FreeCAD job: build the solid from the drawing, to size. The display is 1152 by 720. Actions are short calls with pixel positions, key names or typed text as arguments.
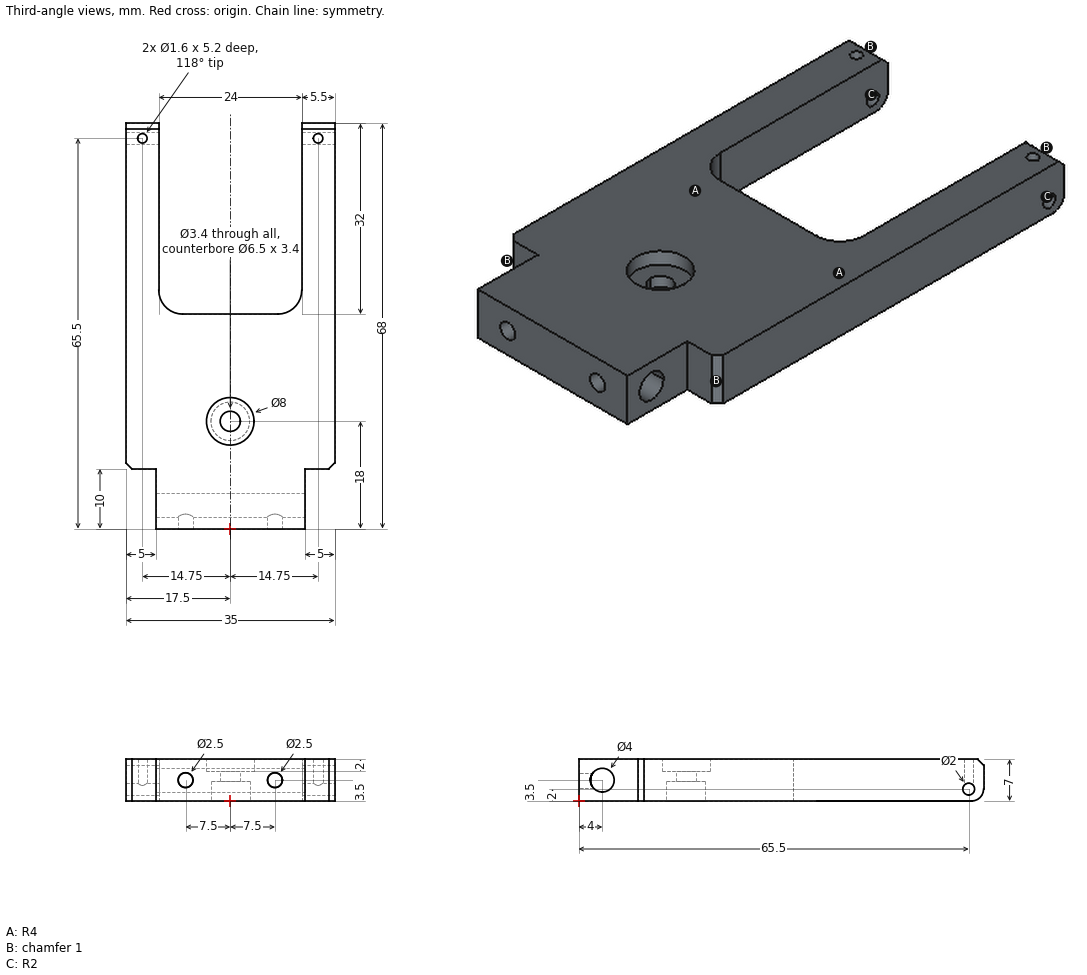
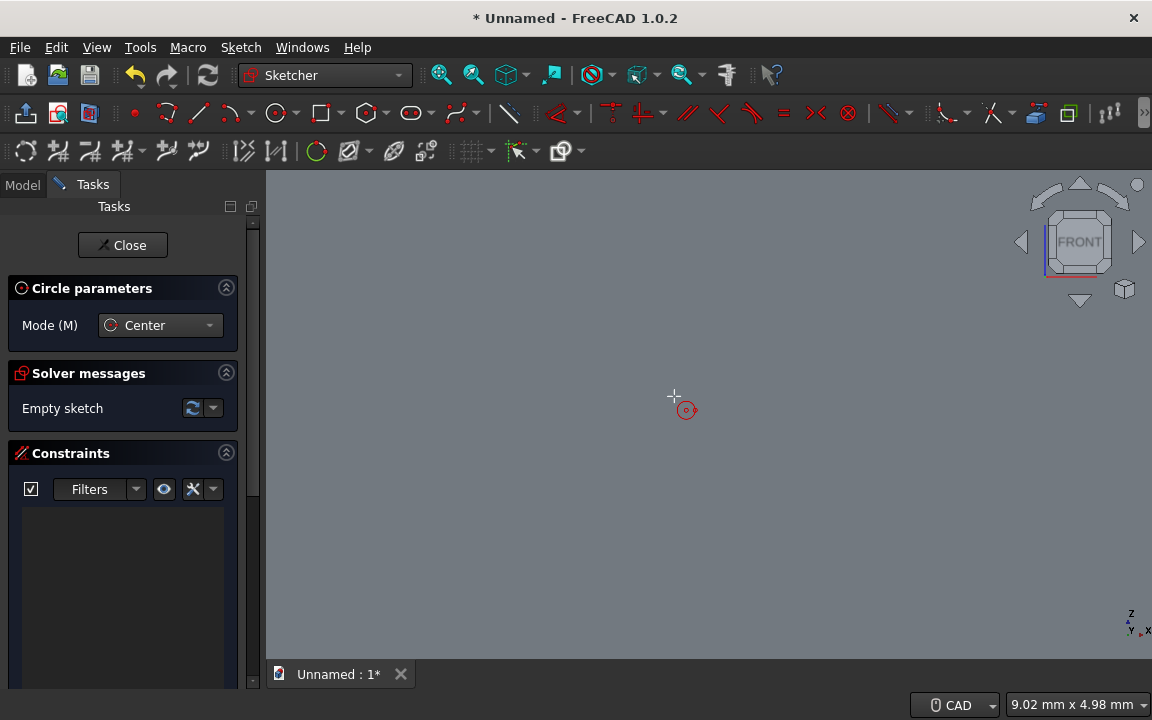
click(632, 415)
move(718, 328)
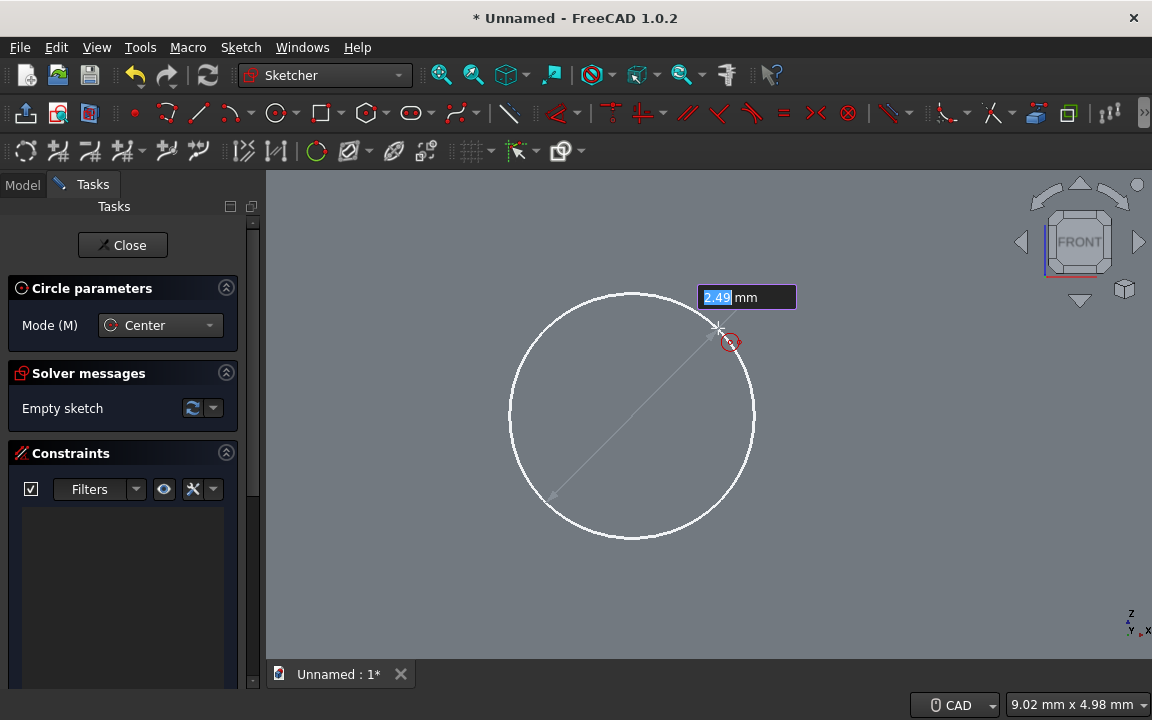
text(2.5)
key(Return)
key(Escape)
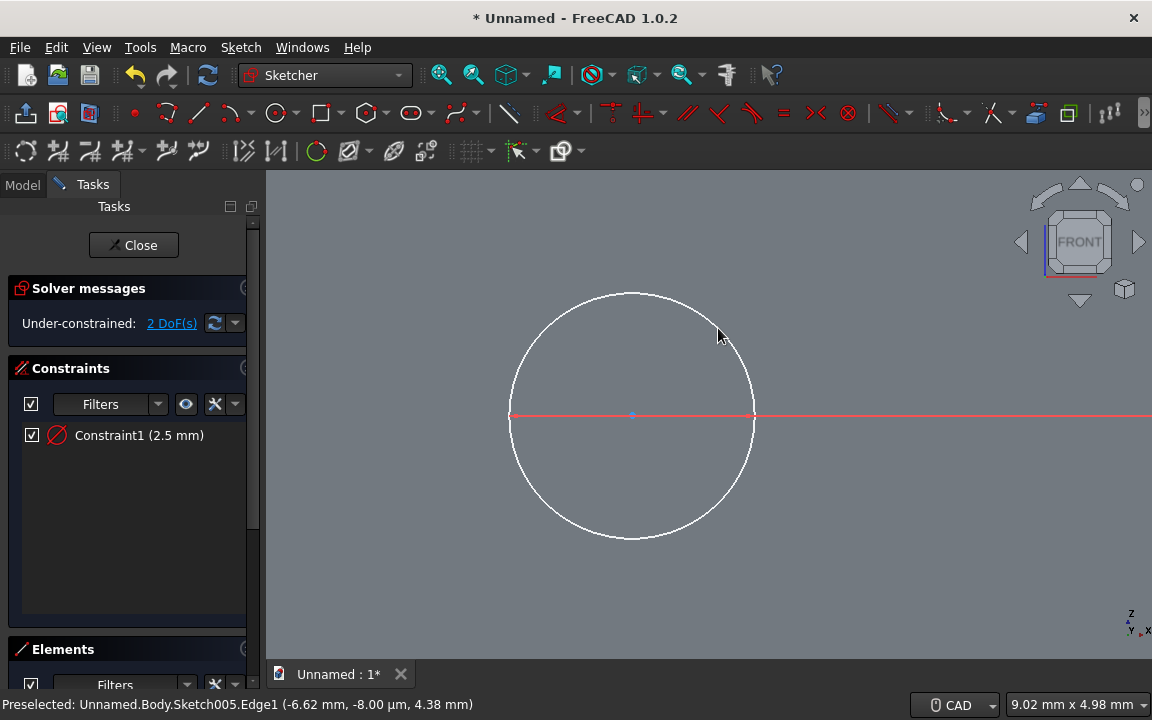
click(556, 114)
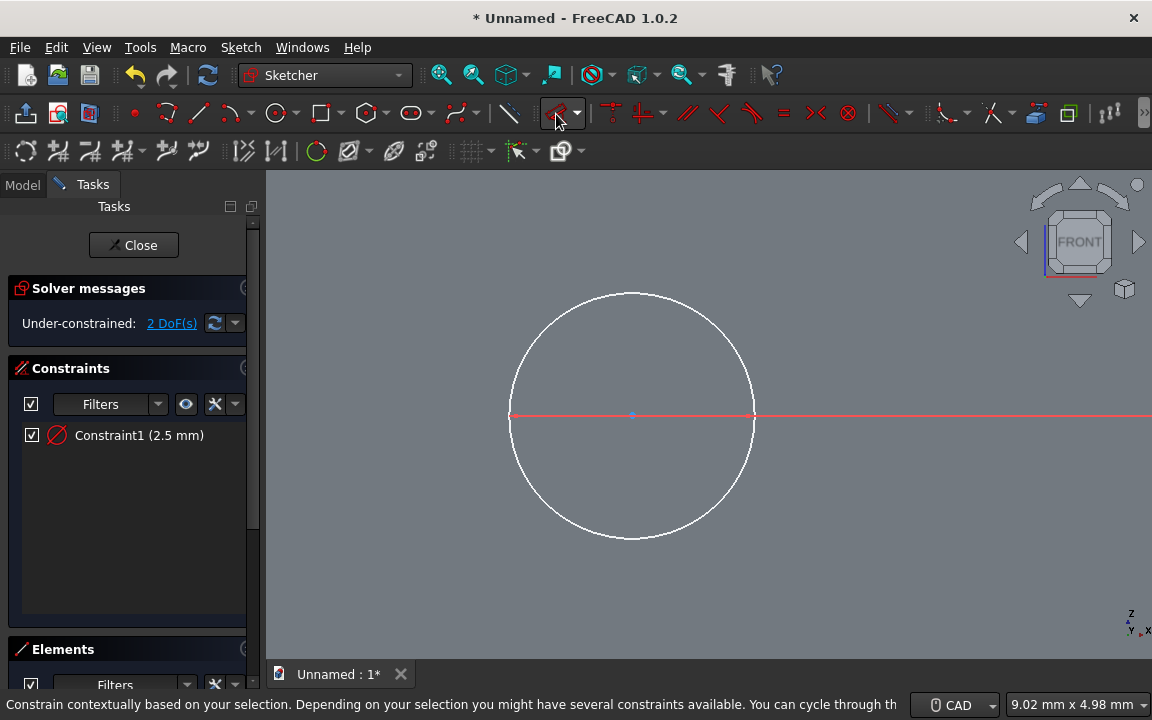
click(632, 416)
click(809, 382)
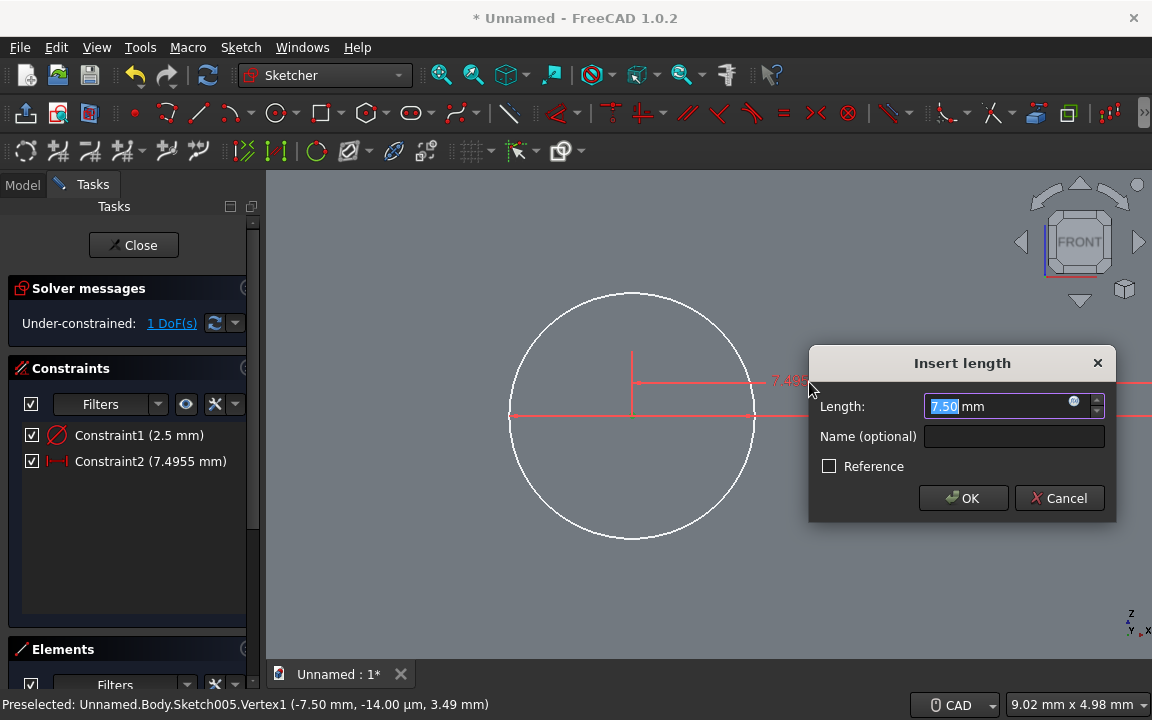
text(7.5)
key(Return)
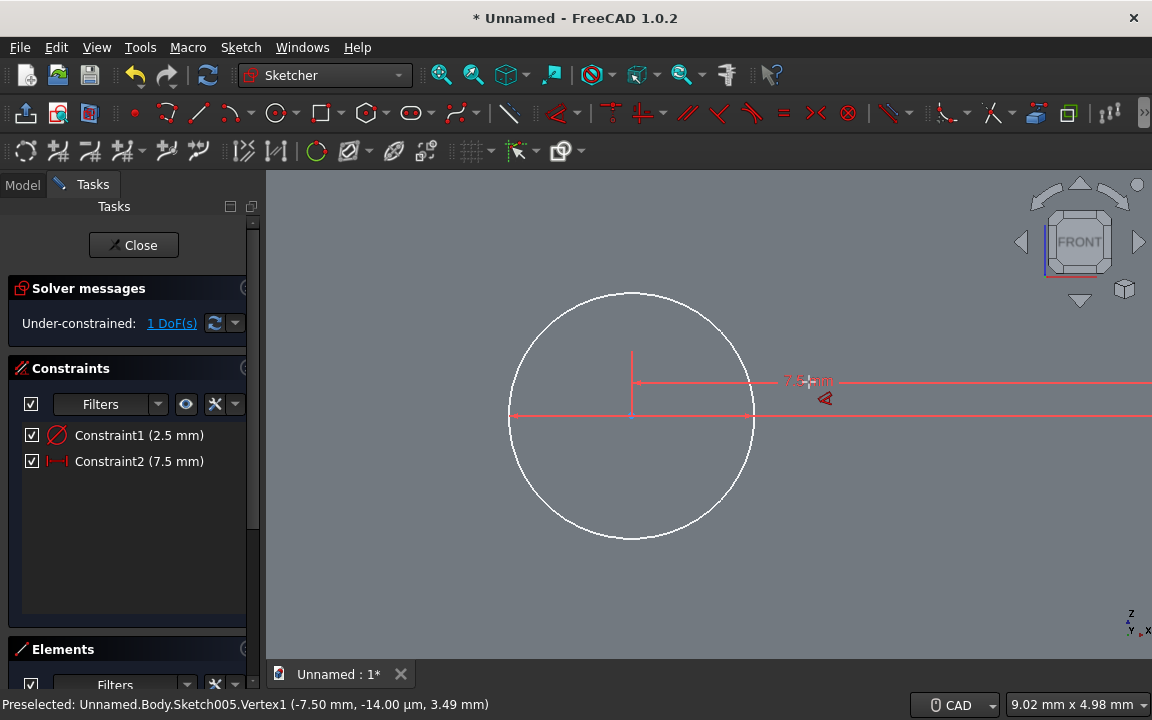
click(632, 416)
click(598, 474)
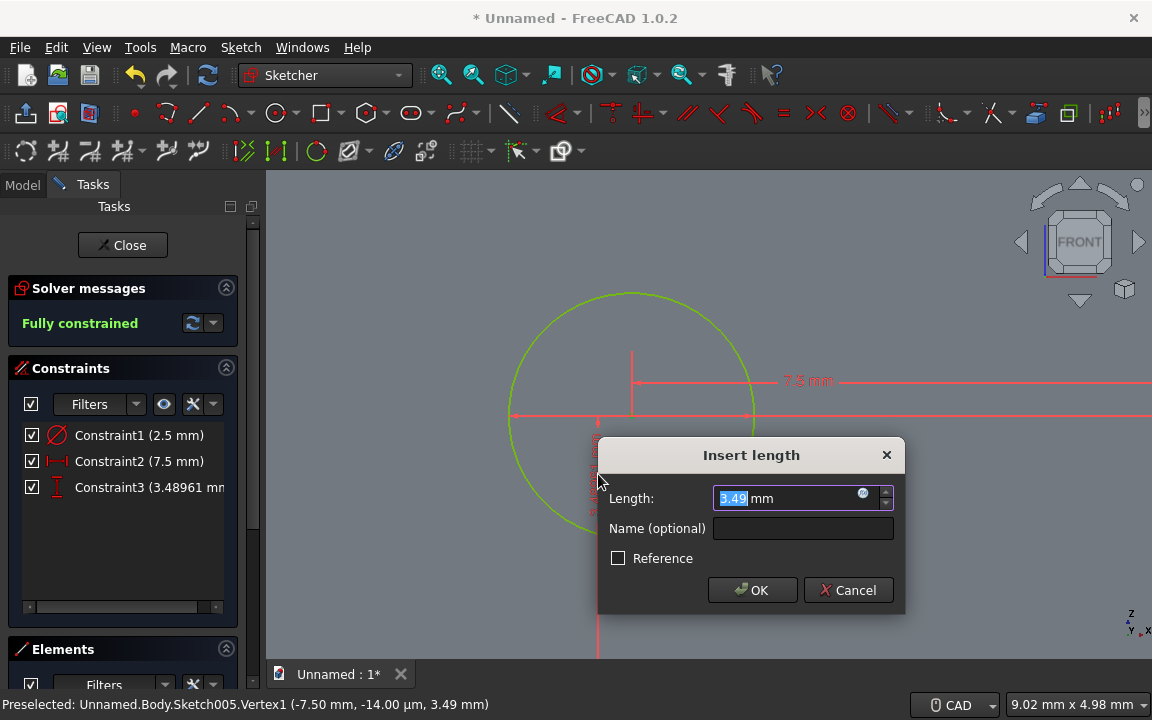
text(3.5)
key(Return)
key(Escape)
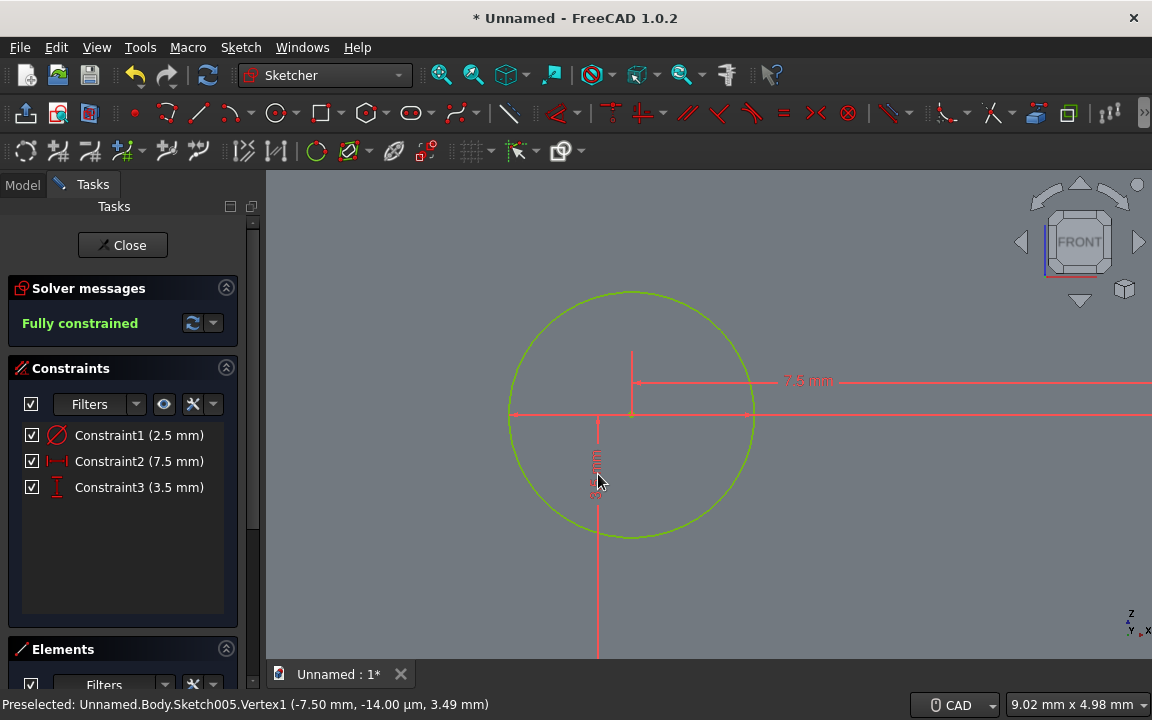
click(123, 245)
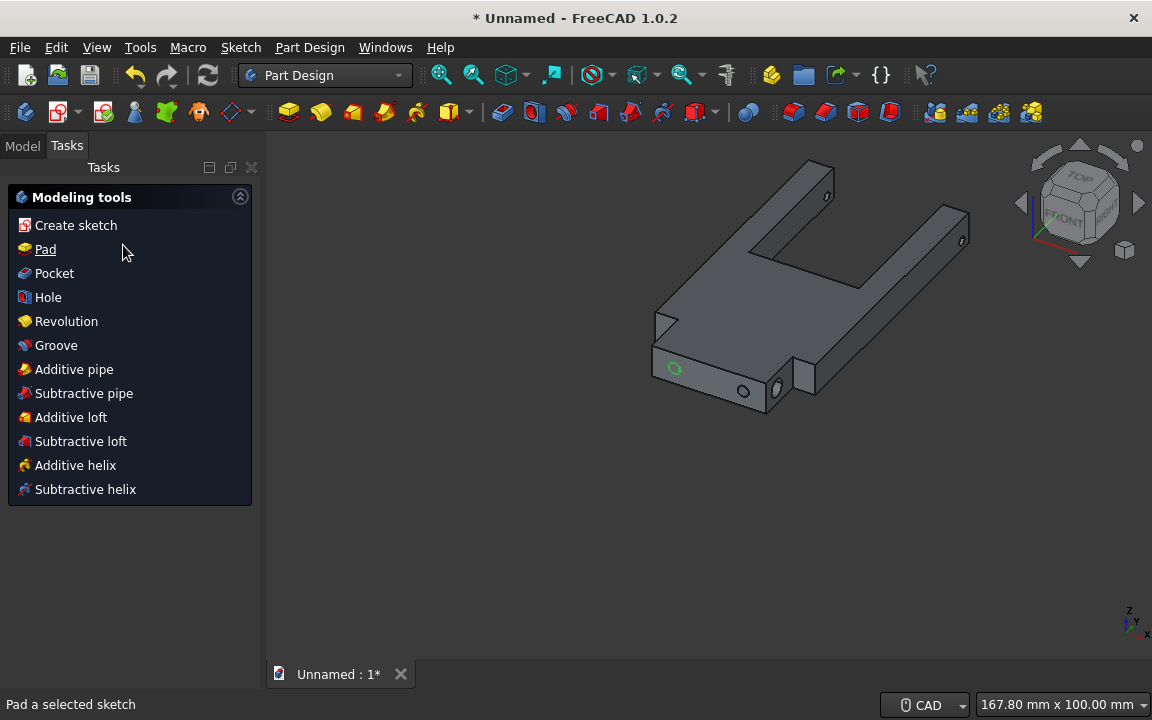
click(504, 112)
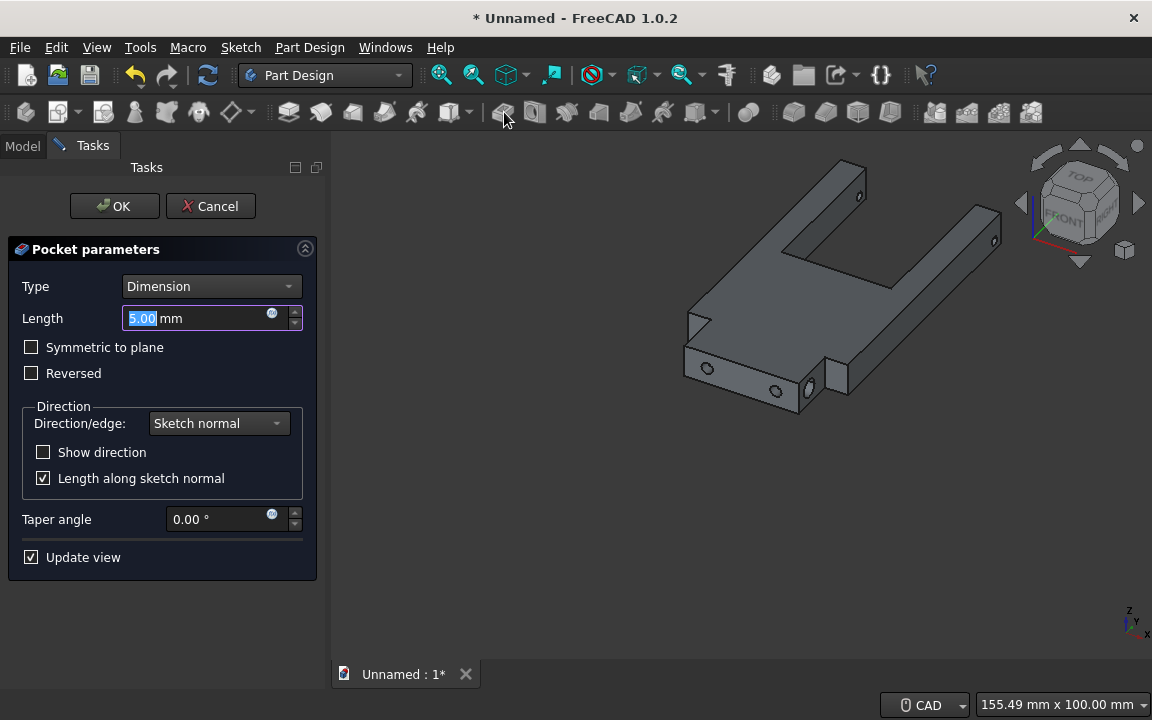
click(212, 286)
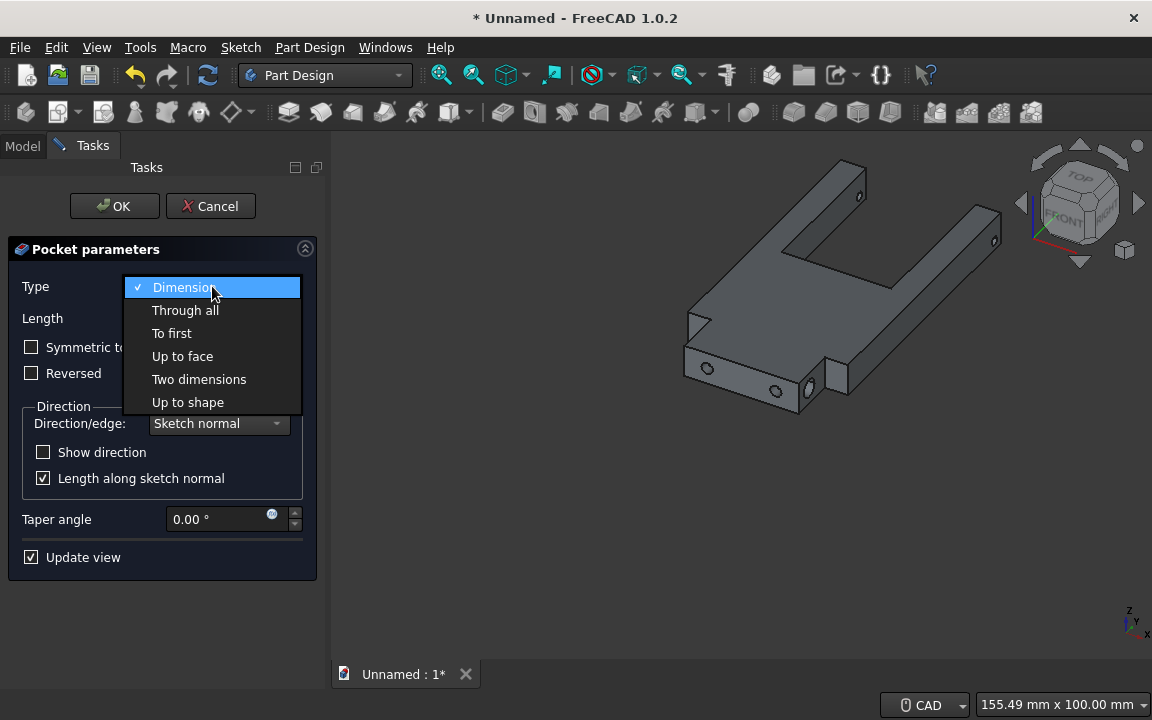
click(212, 334)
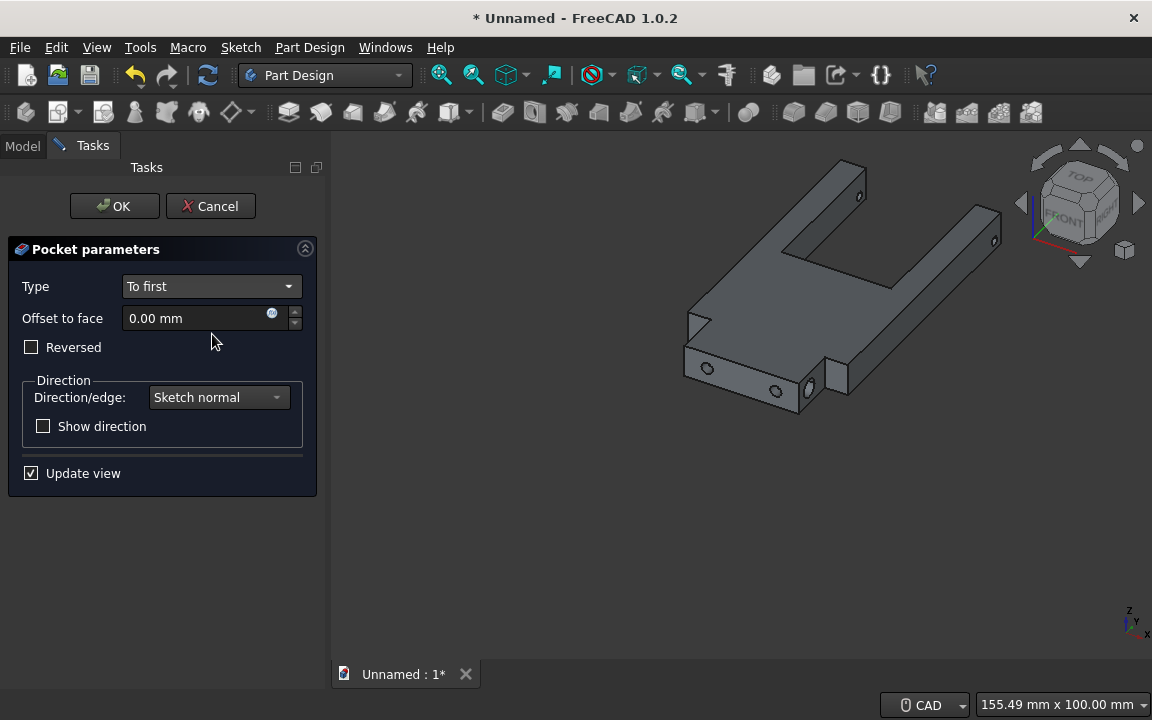
click(115, 206)